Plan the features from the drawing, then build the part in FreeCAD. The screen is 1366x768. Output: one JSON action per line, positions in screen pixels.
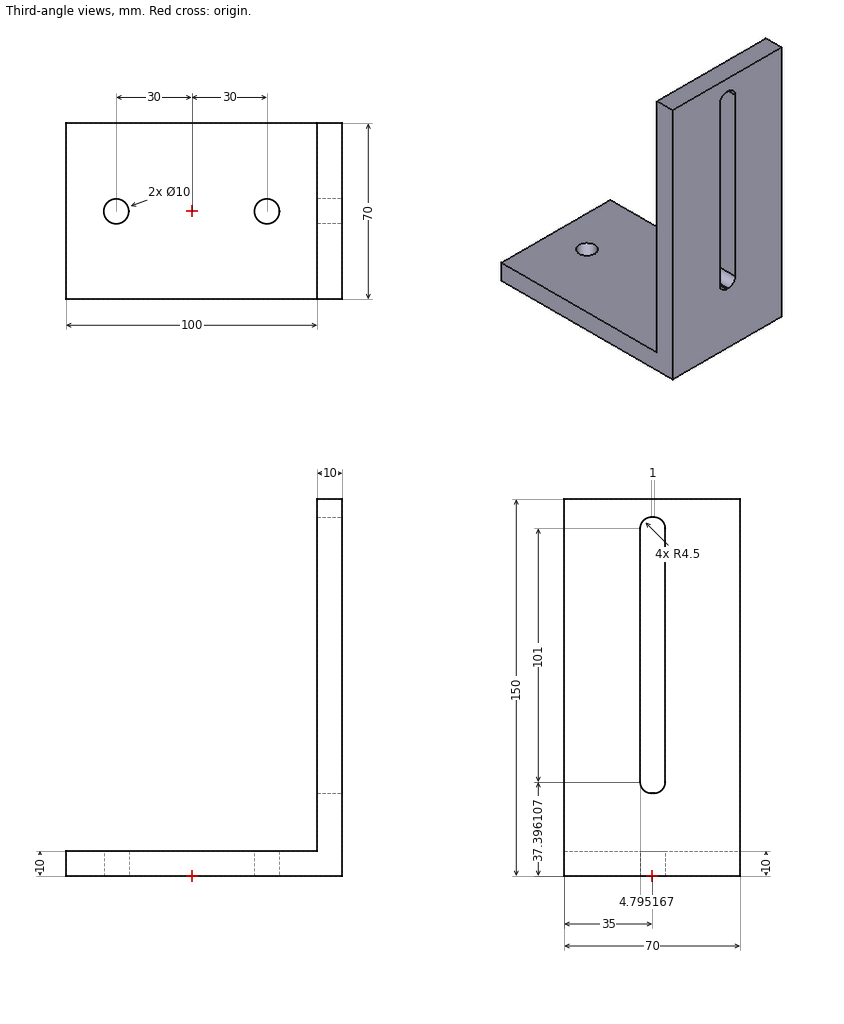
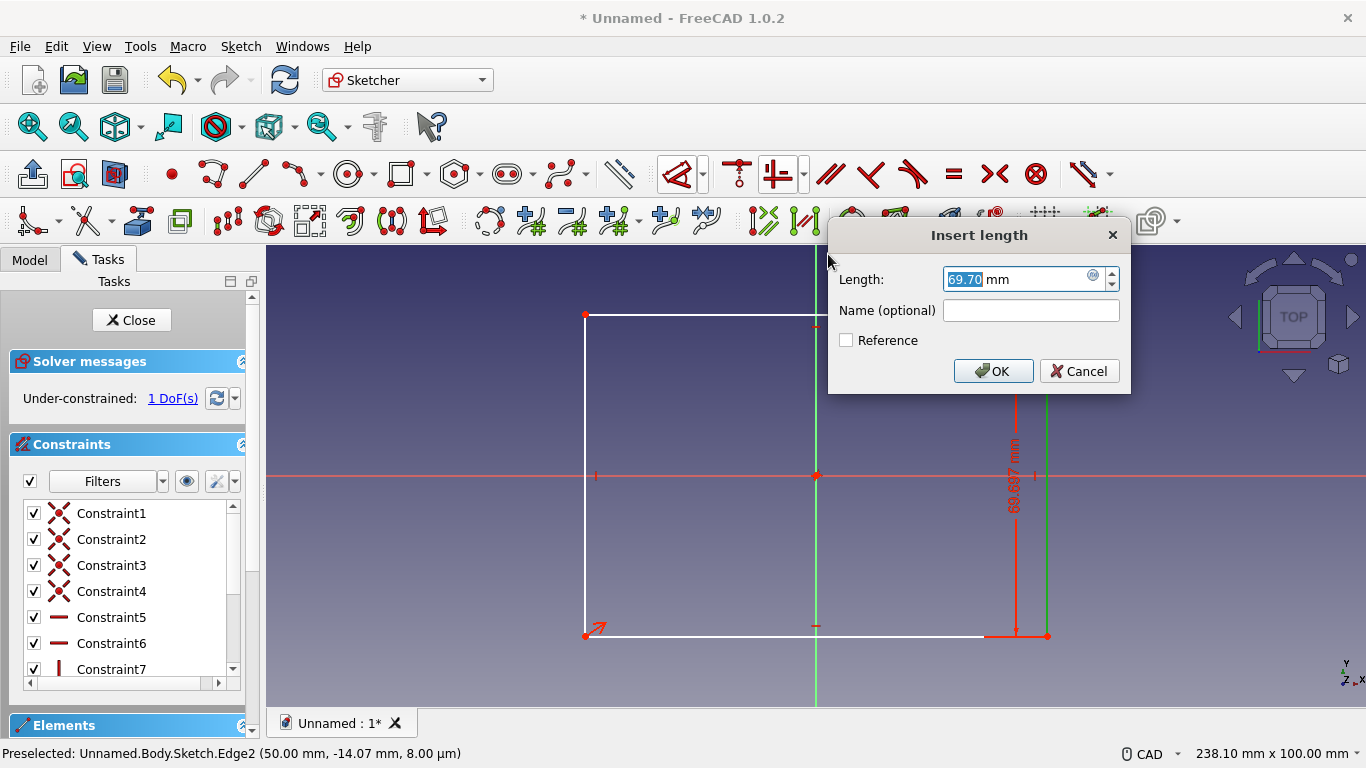
{"action": "type", "text": "70"}
{"action": "key", "text": "Return"}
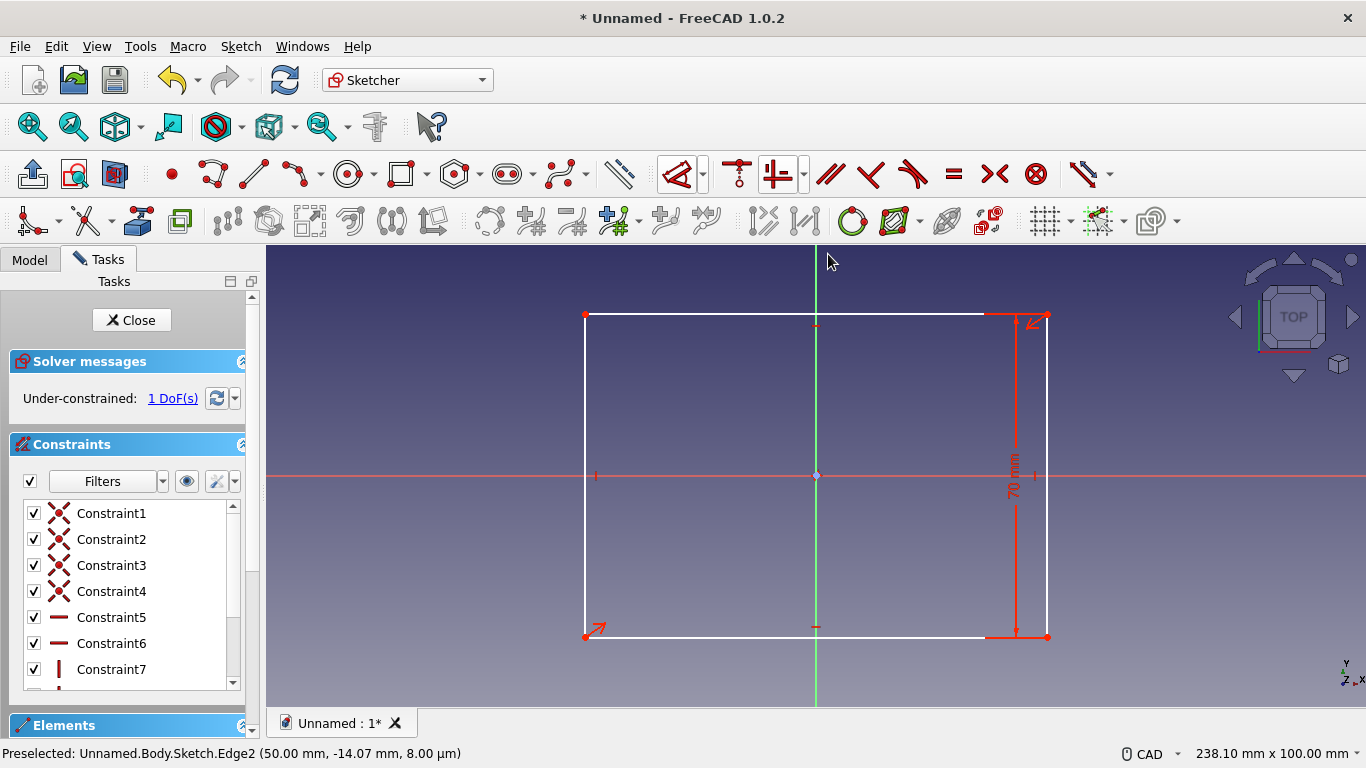
{"action": "left_click", "coordinate": [724, 638]}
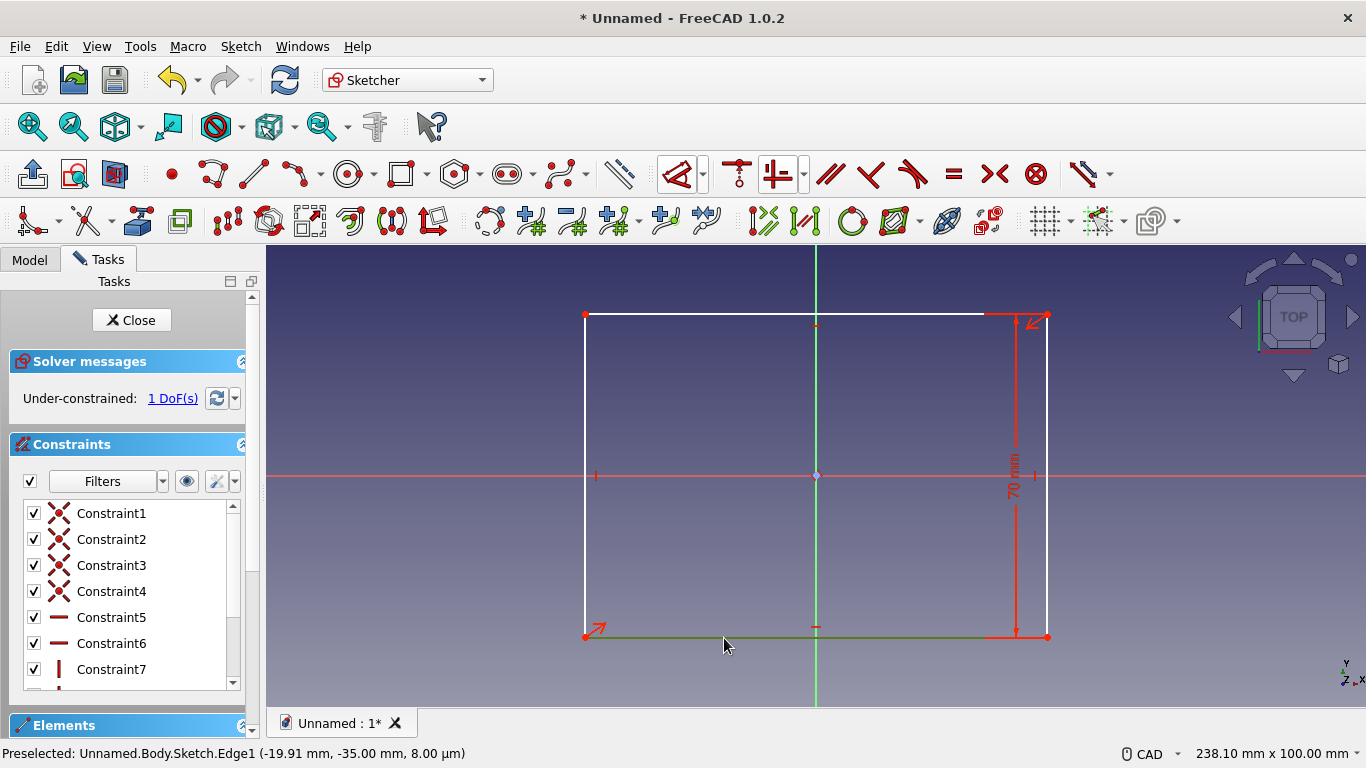
{"action": "left_click", "coordinate": [702, 174]}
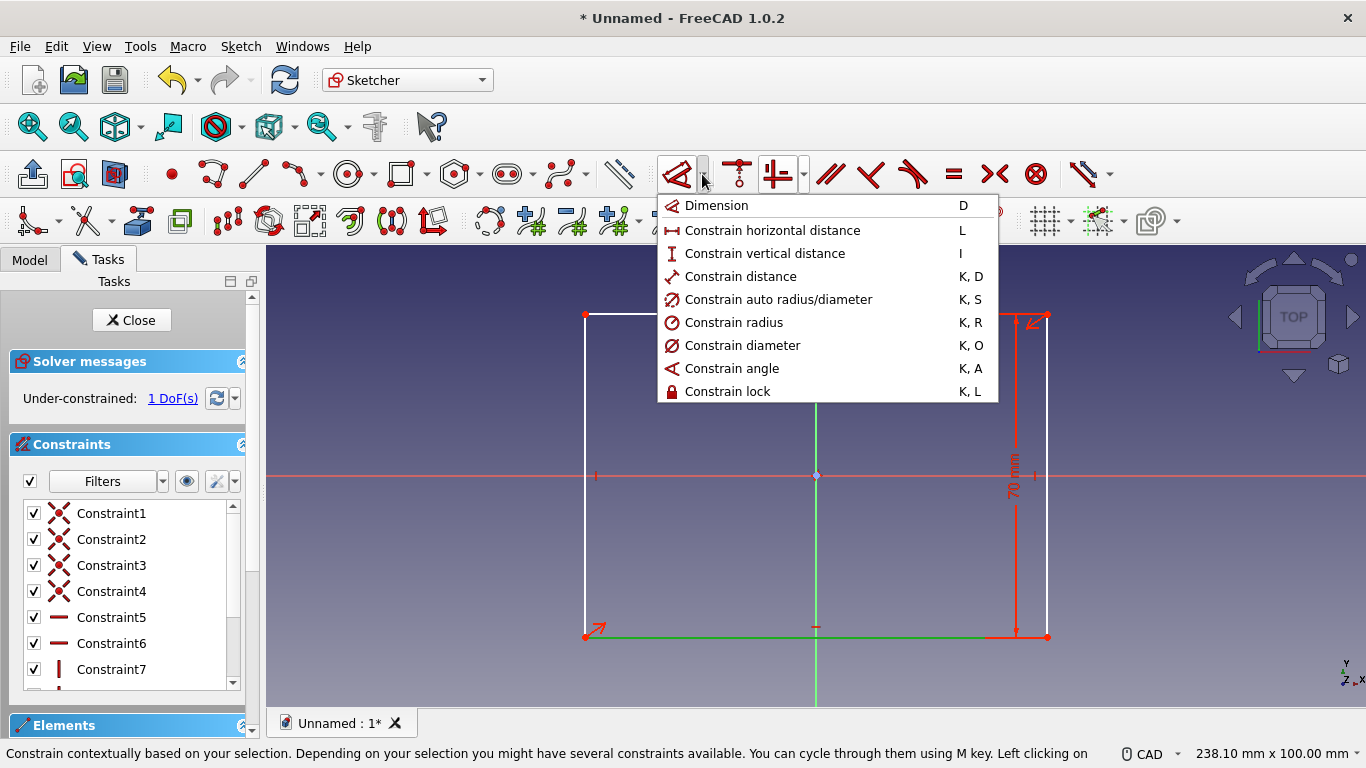
{"action": "left_click", "coordinate": [828, 230]}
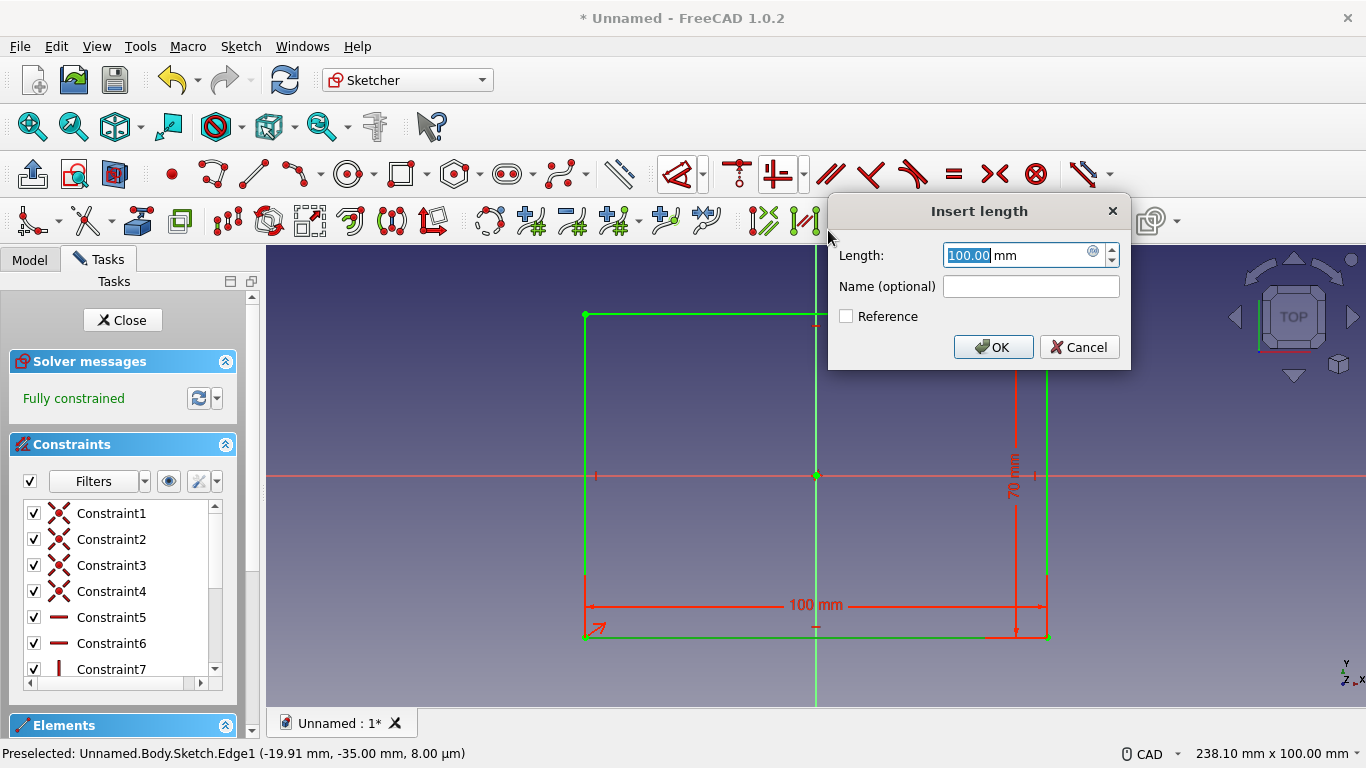
{"action": "type", "text": "100"}
{"action": "key", "text": "Return"}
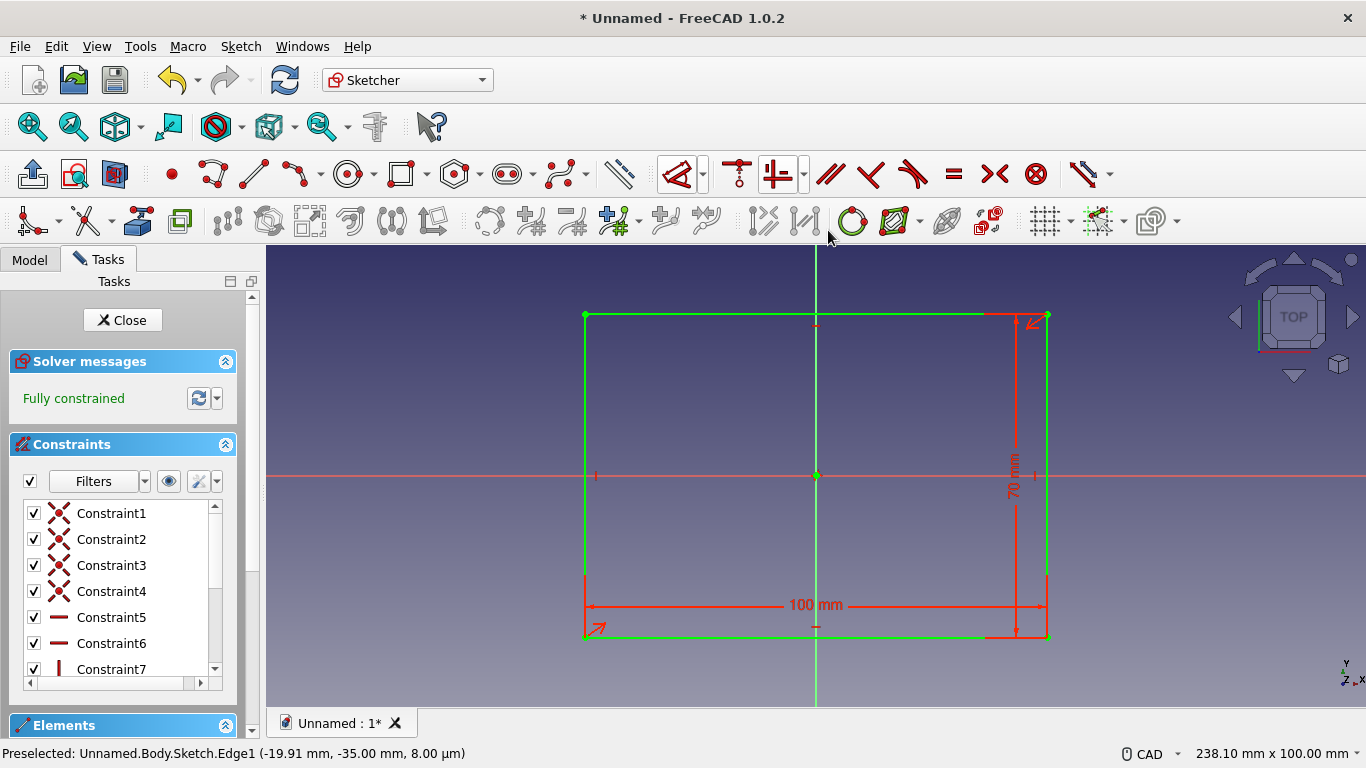
{"action": "left_click", "coordinate": [123, 320]}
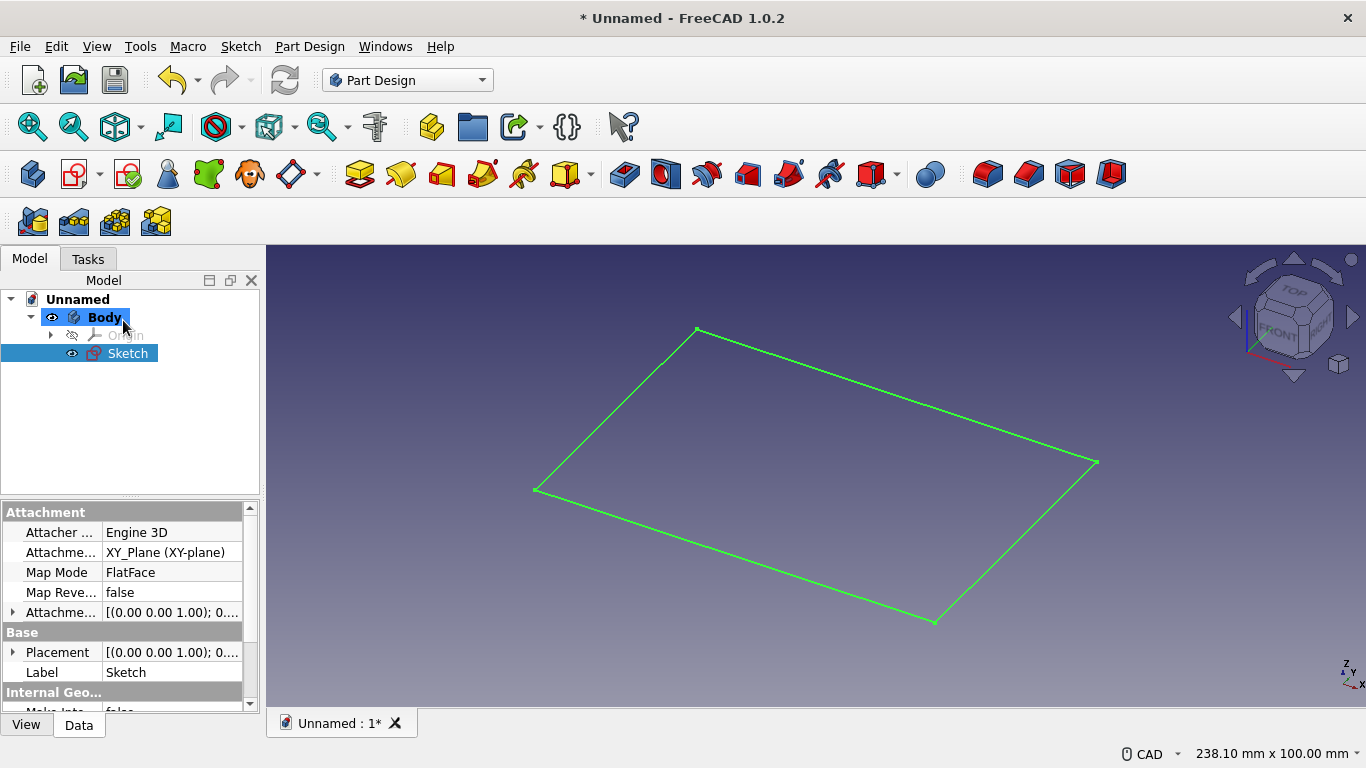
{"action": "left_click", "coordinate": [360, 174]}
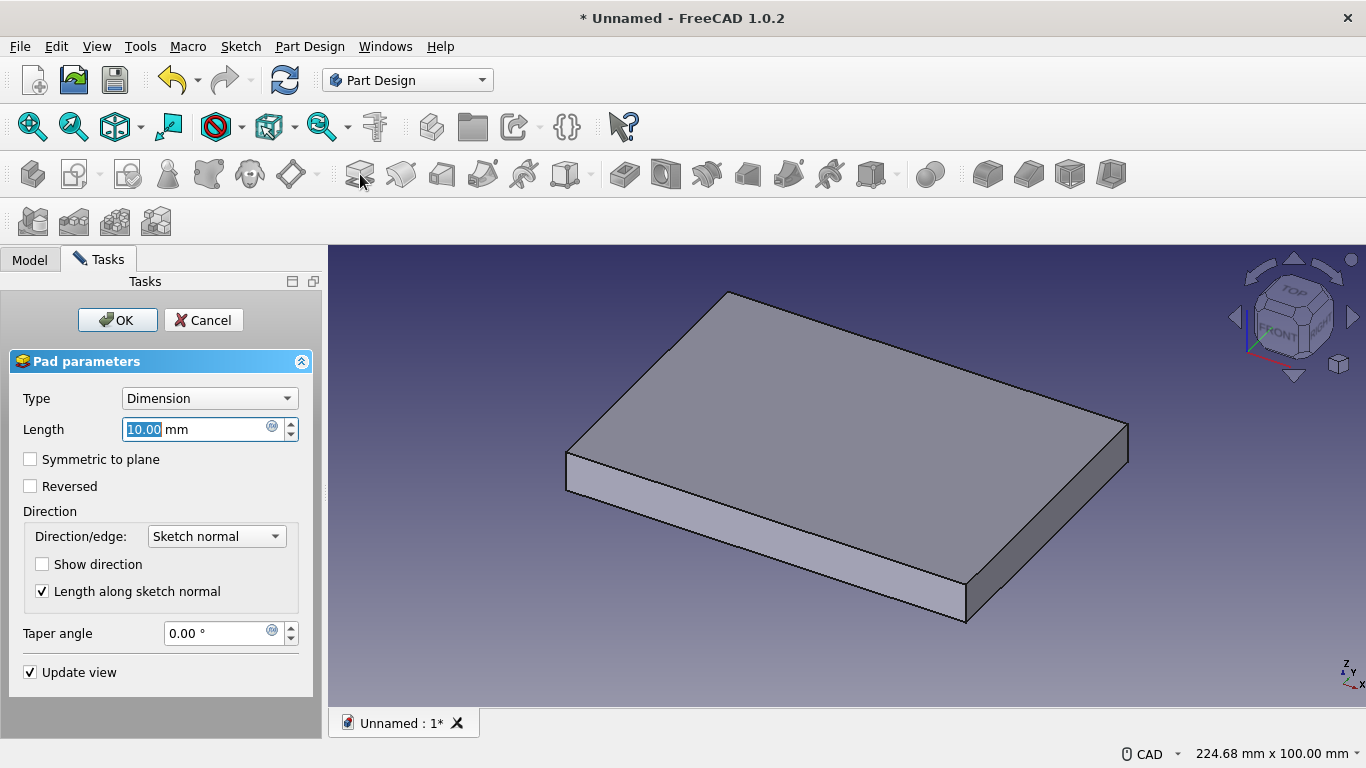
{"action": "type", "text": "10"}
{"action": "key", "text": "Tab"}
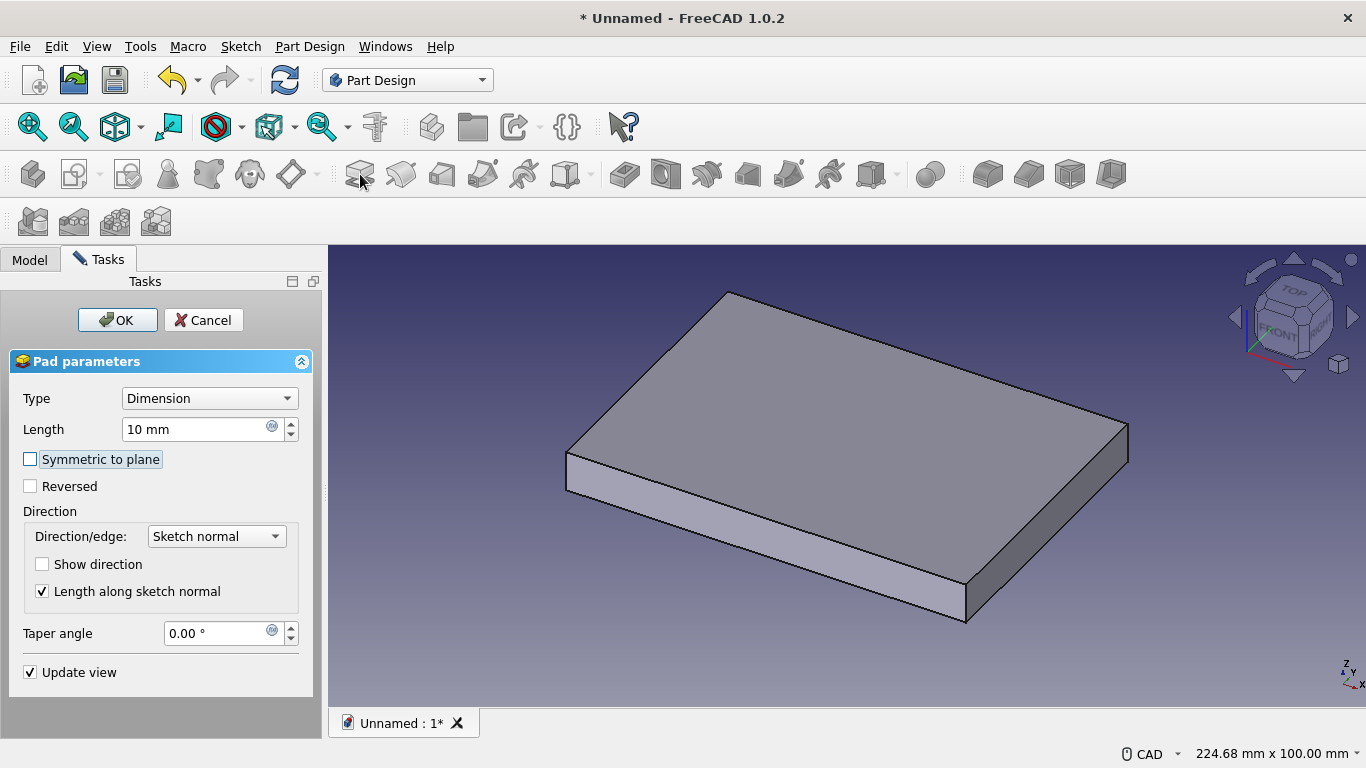
{"action": "left_click", "coordinate": [118, 320]}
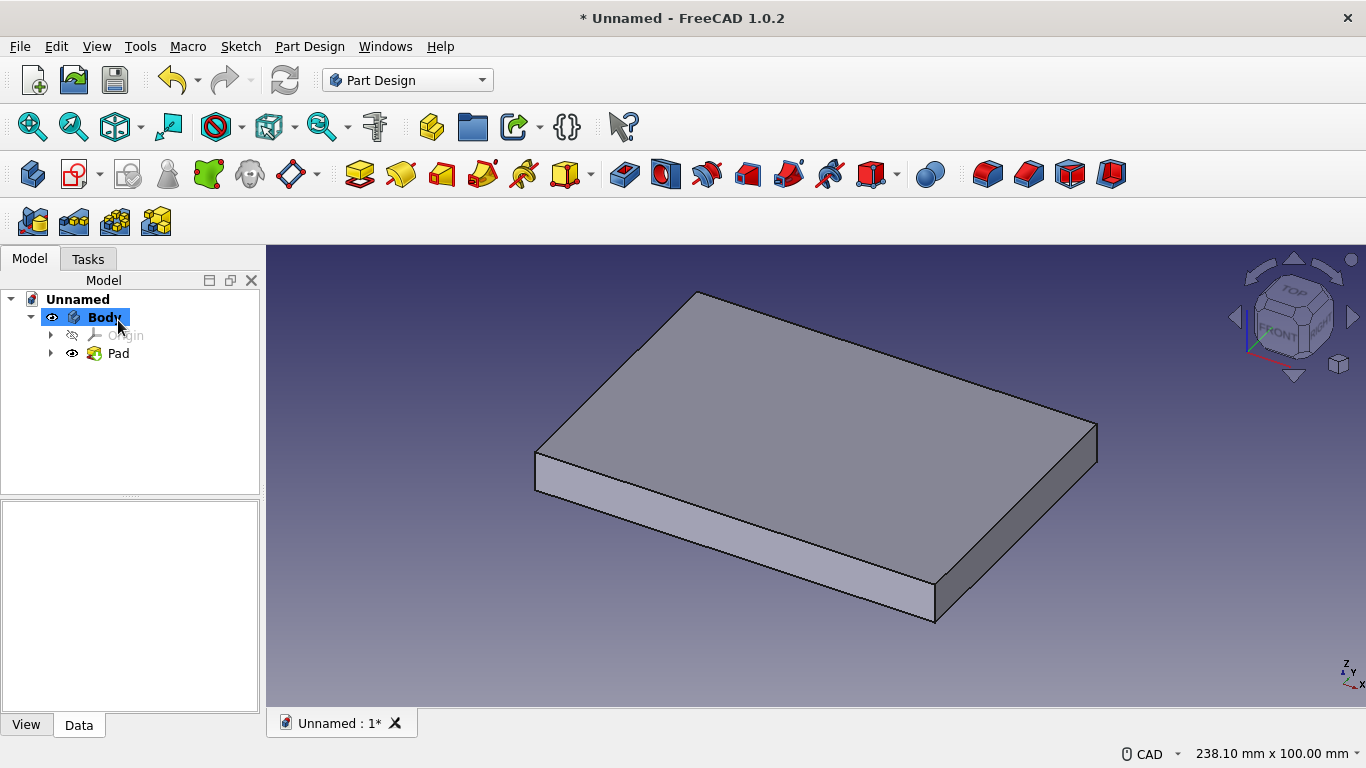
{"action": "left_click", "coordinate": [873, 456]}